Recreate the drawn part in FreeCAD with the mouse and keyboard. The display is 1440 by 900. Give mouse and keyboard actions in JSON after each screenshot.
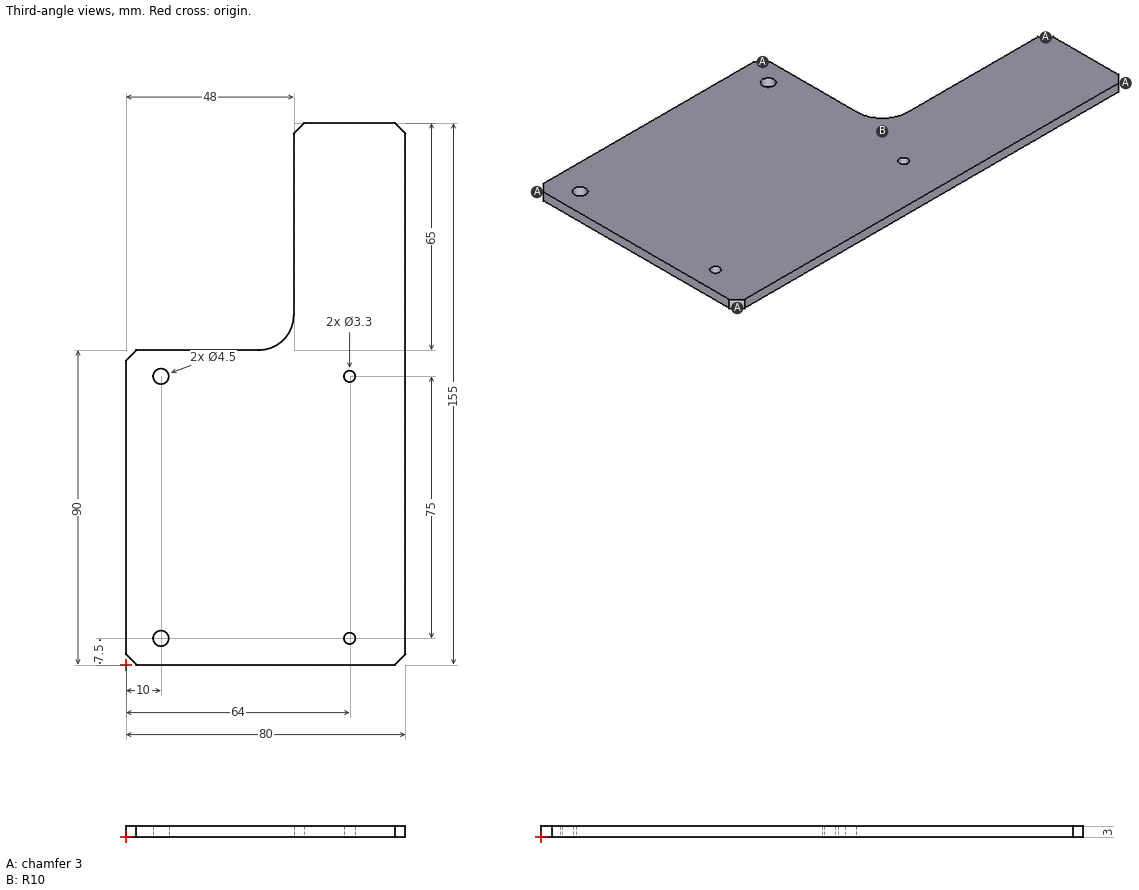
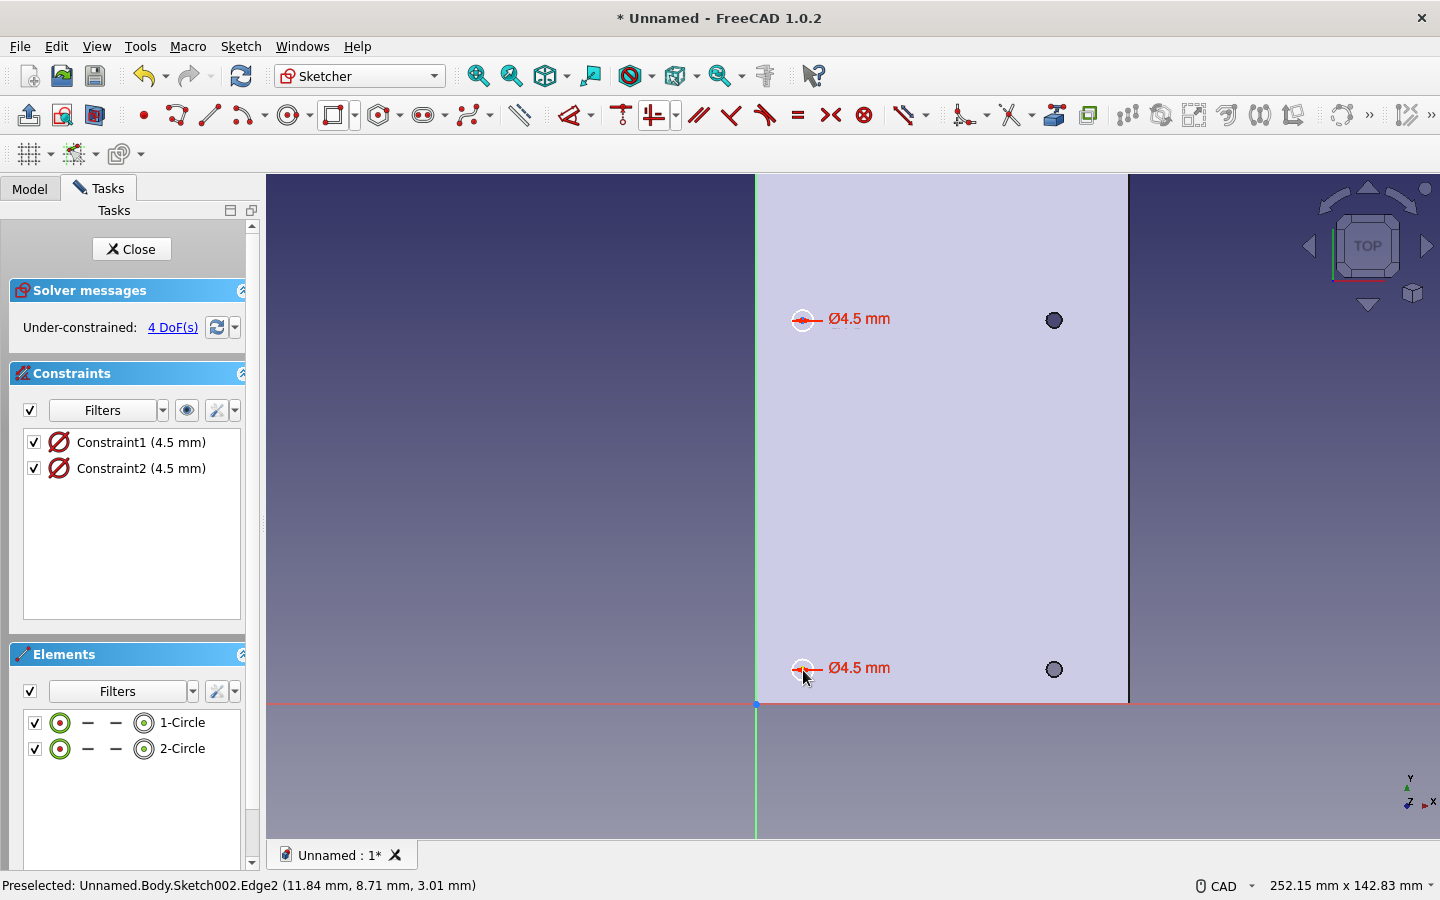
{"action": "left_click", "coordinate": [803, 321]}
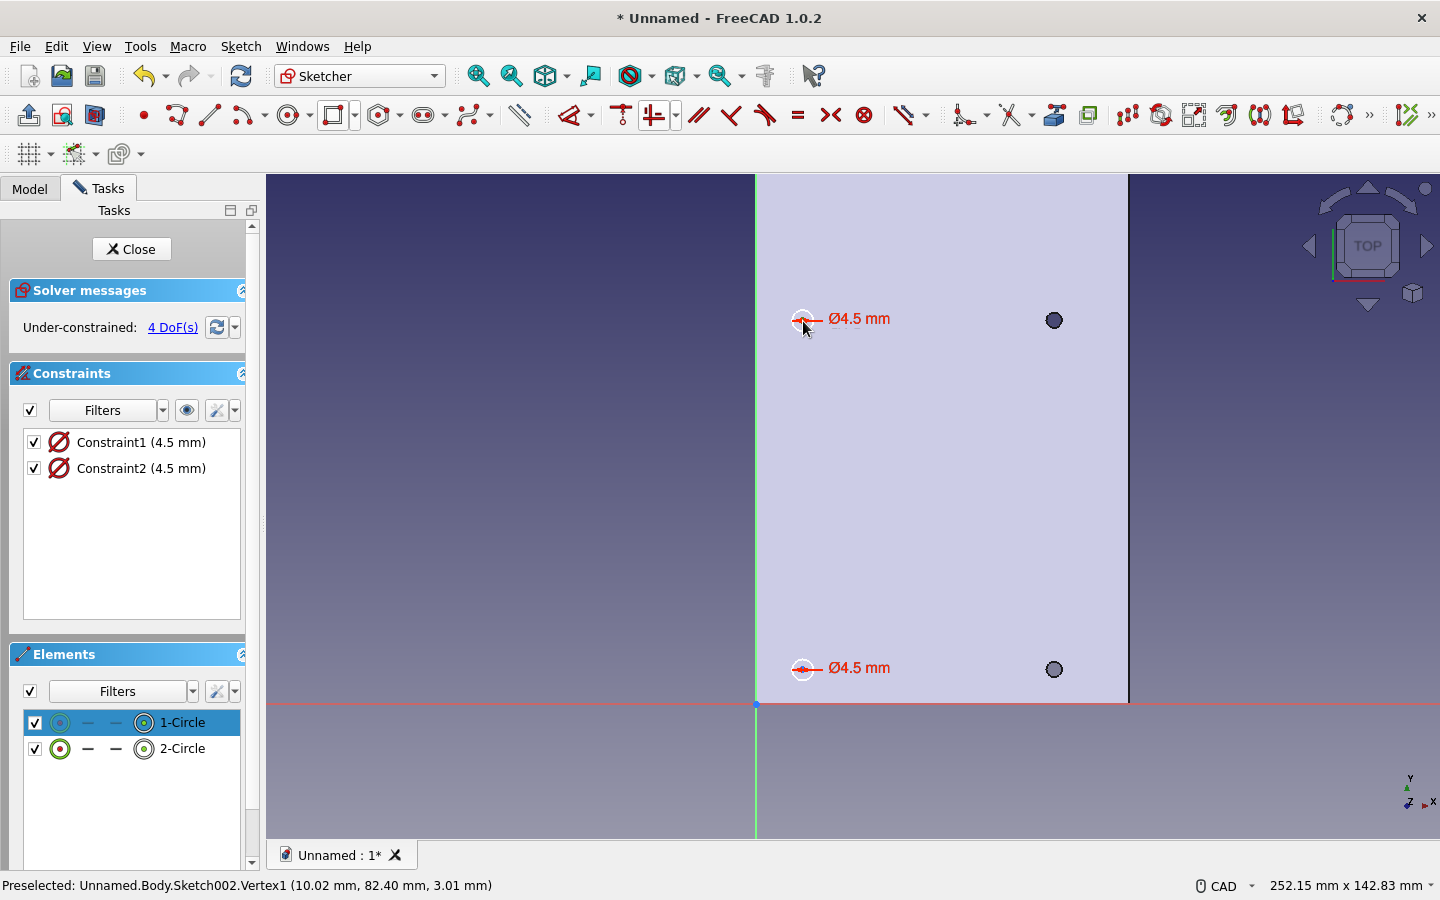
{"action": "left_click", "coordinate": [803, 670]}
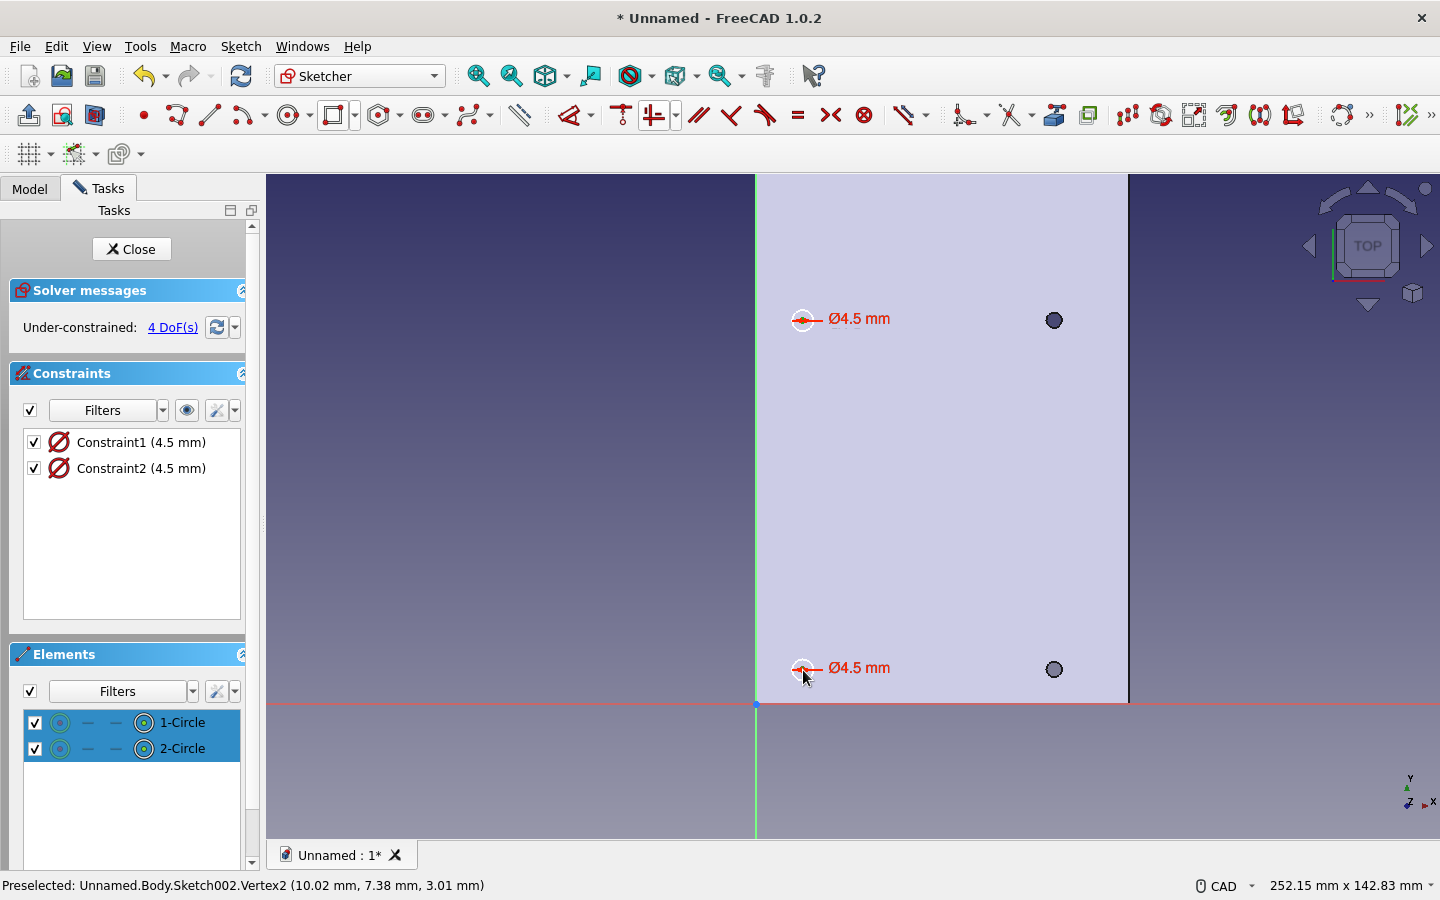
{"action": "key", "text": "v"}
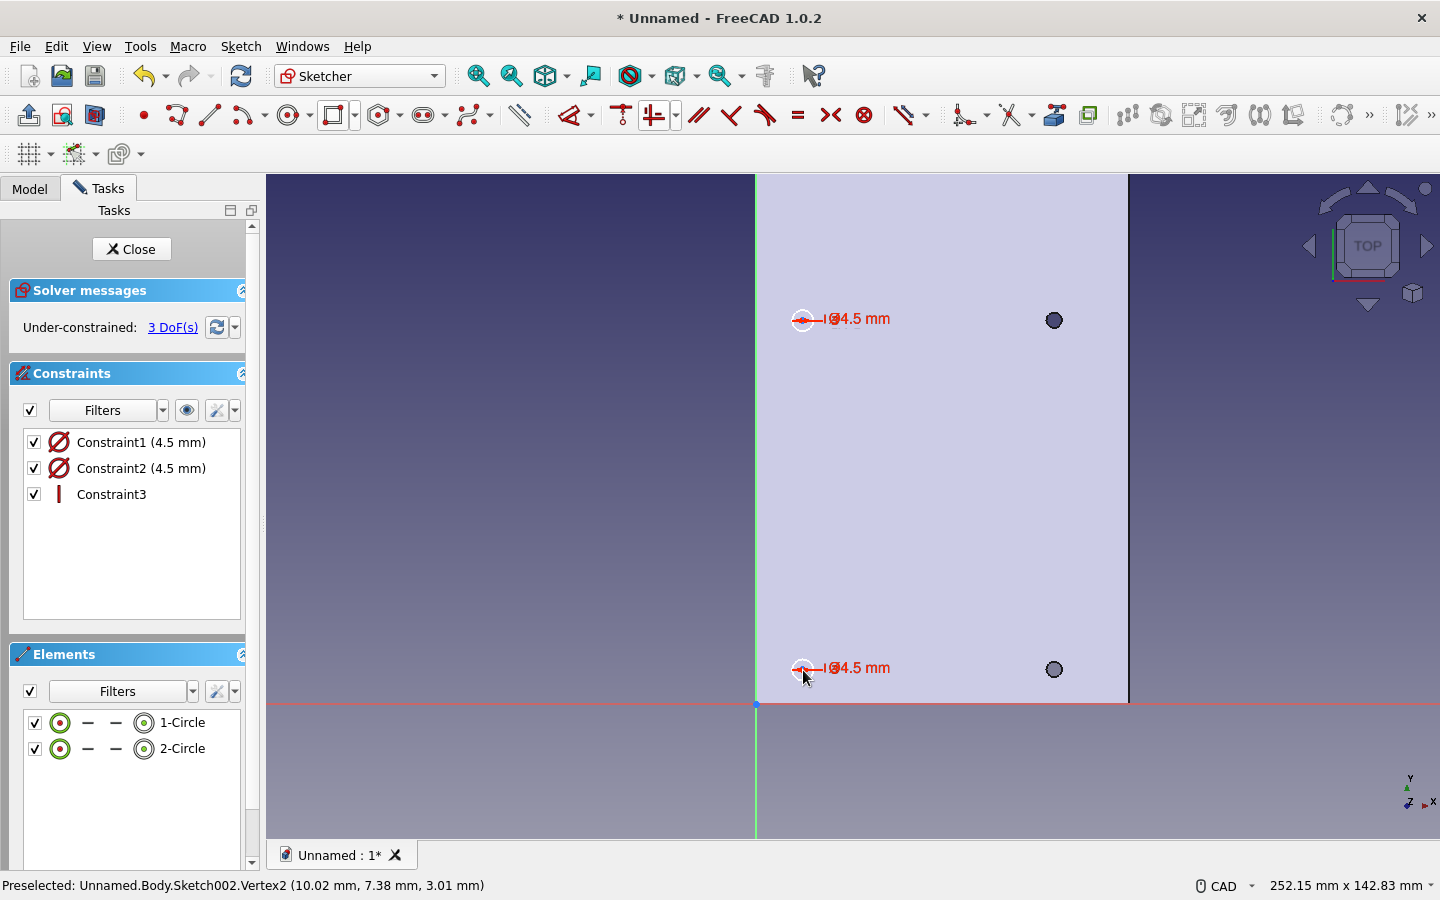
{"action": "key", "text": "d"}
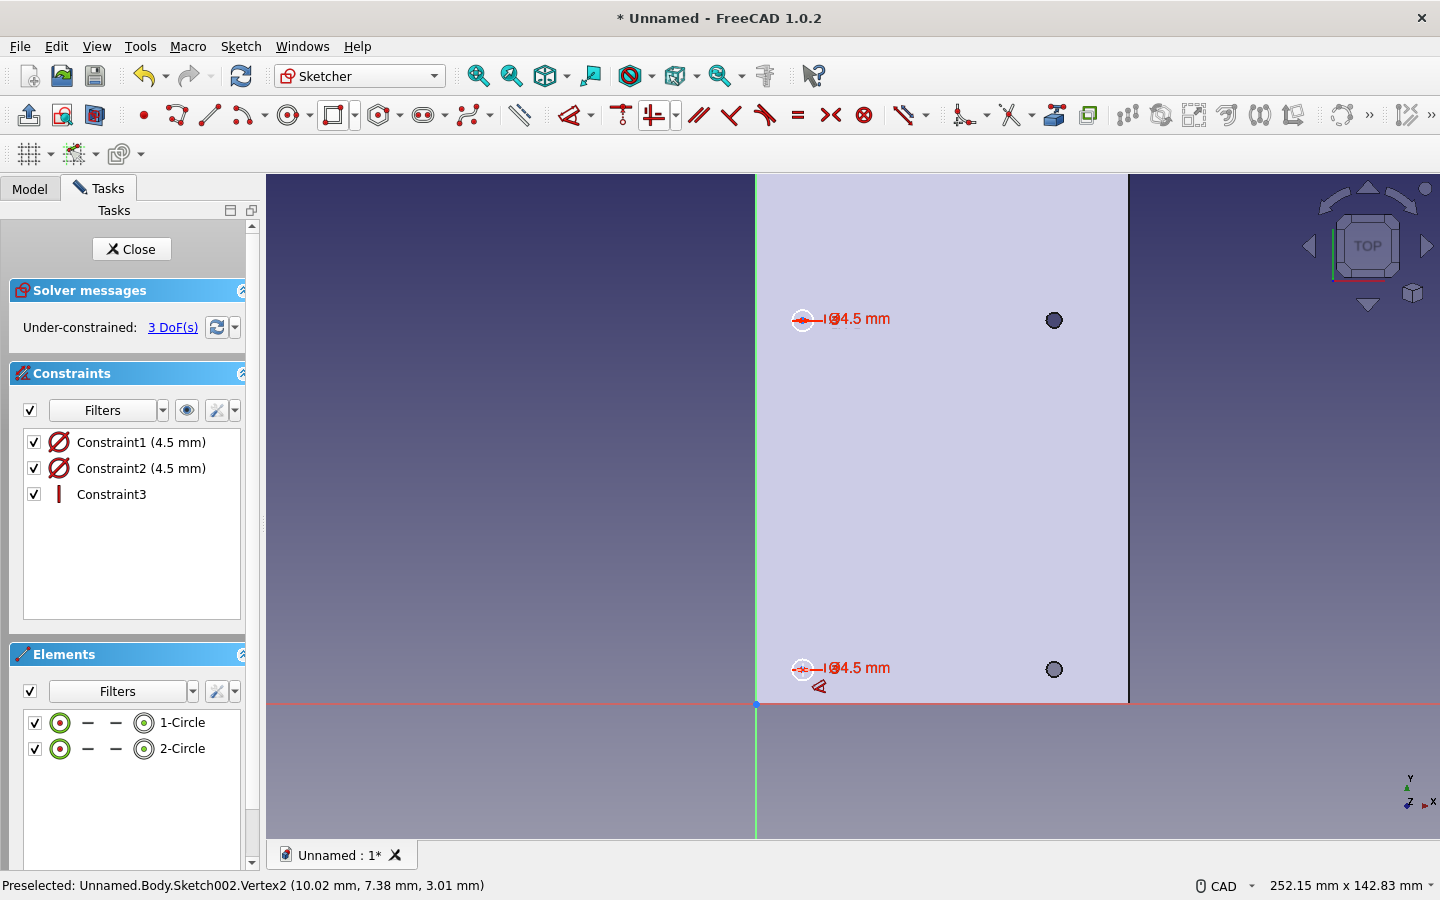
{"action": "left_click", "coordinate": [803, 321]}
{"action": "left_click", "coordinate": [779, 738]}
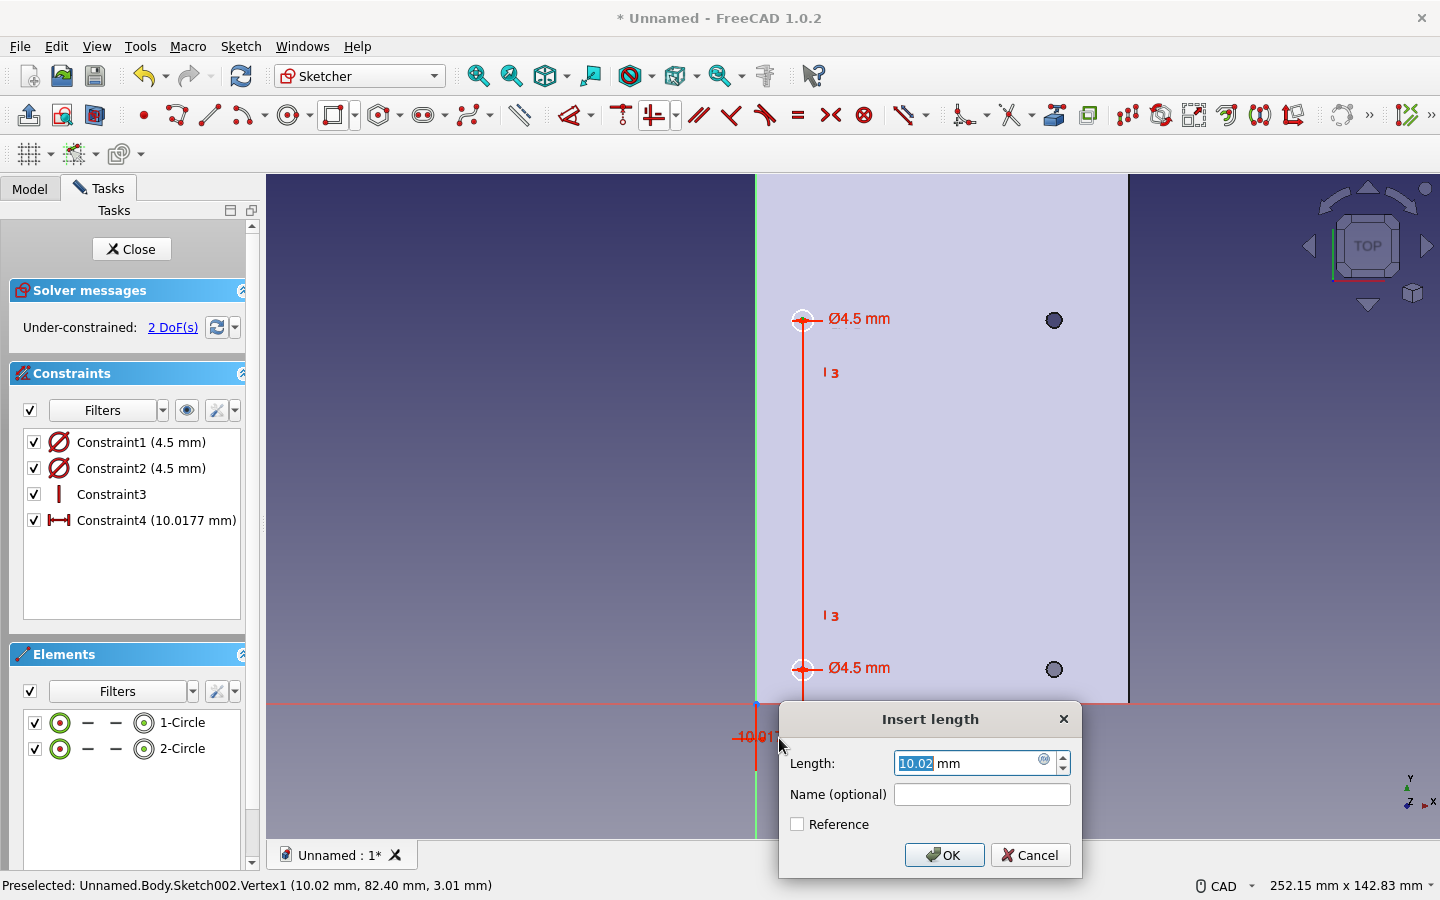
{"action": "type", "text": "10"}
{"action": "key", "text": "Return"}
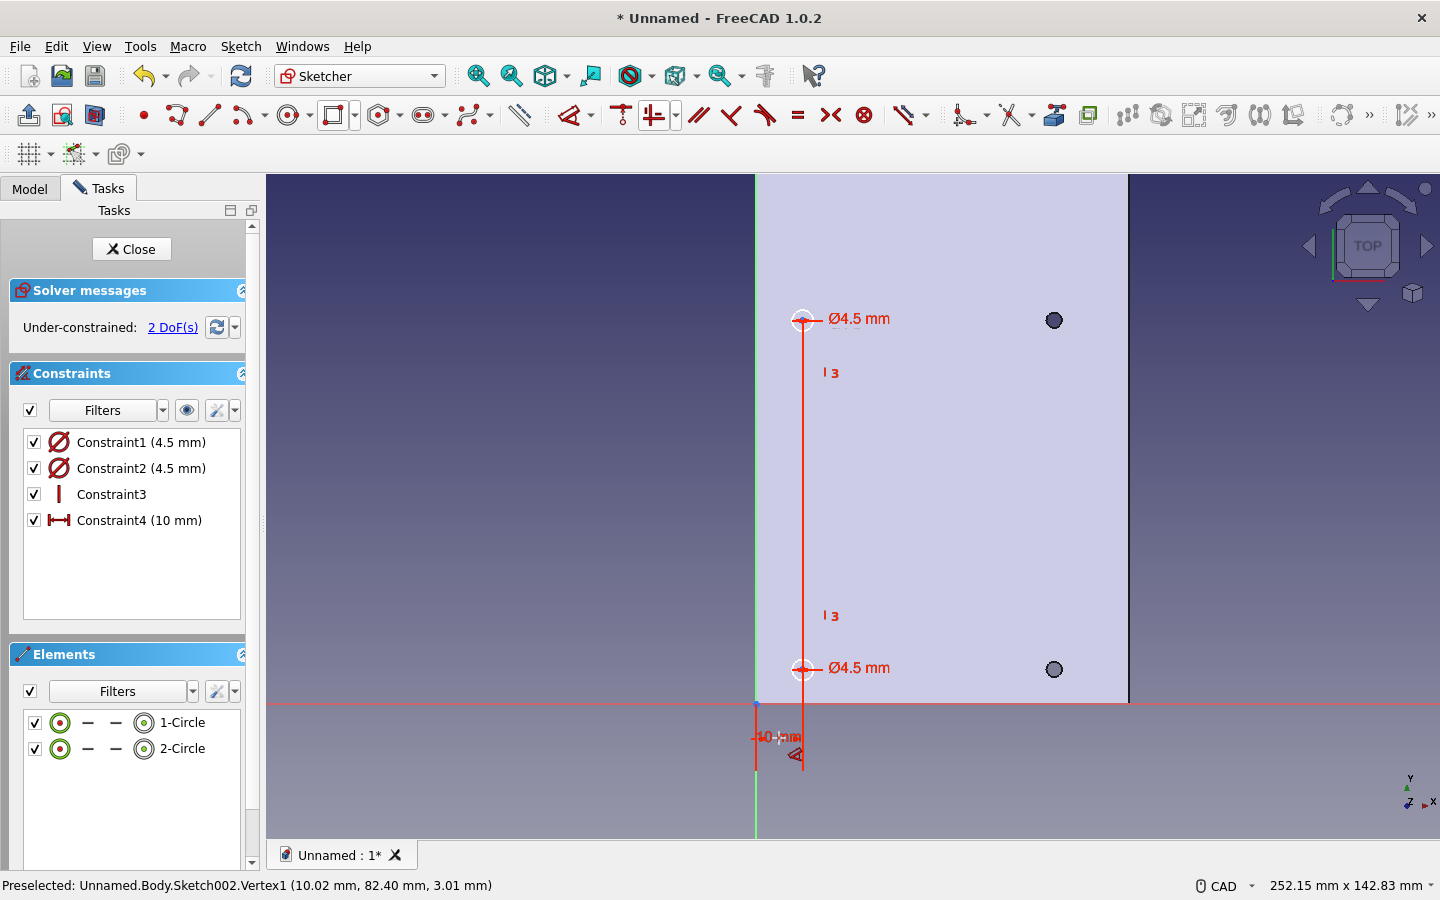
{"action": "left_click", "coordinate": [803, 670]}
{"action": "left_click", "coordinate": [722, 687]}